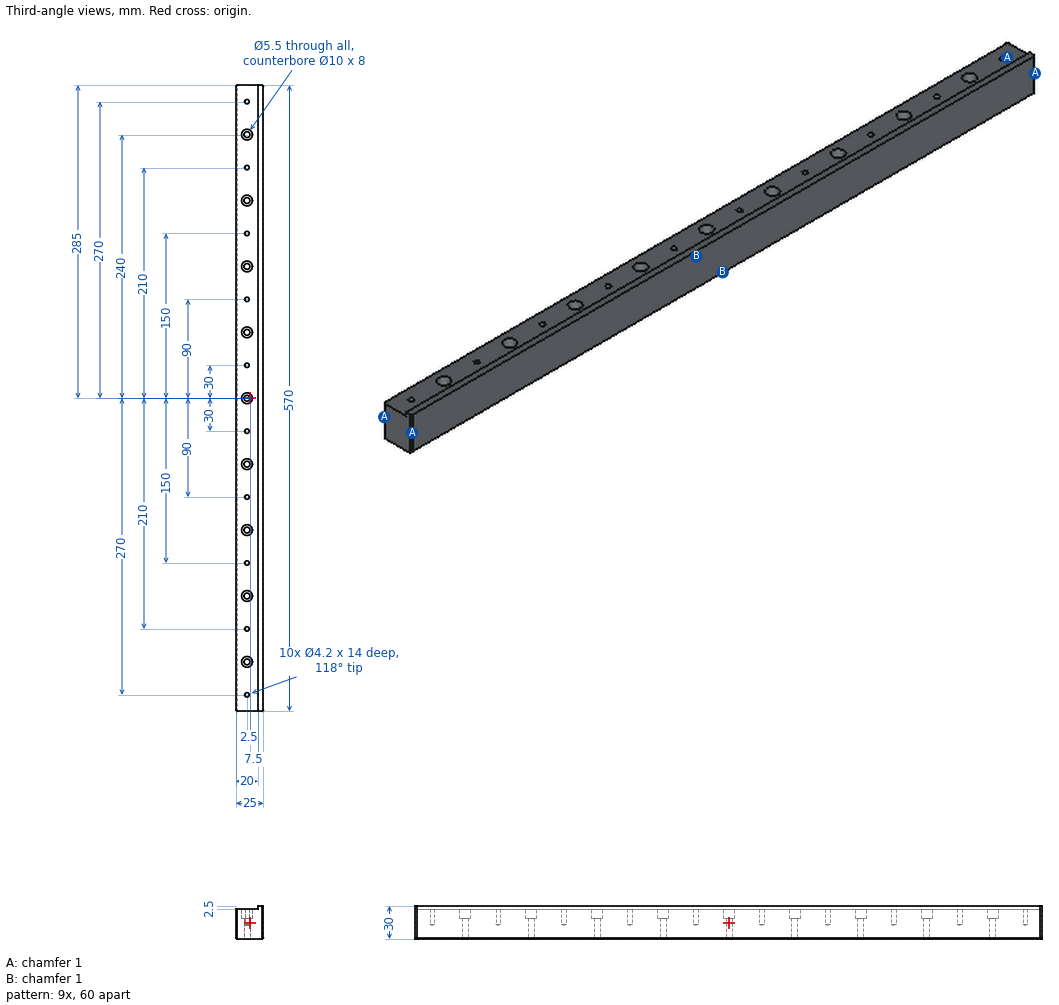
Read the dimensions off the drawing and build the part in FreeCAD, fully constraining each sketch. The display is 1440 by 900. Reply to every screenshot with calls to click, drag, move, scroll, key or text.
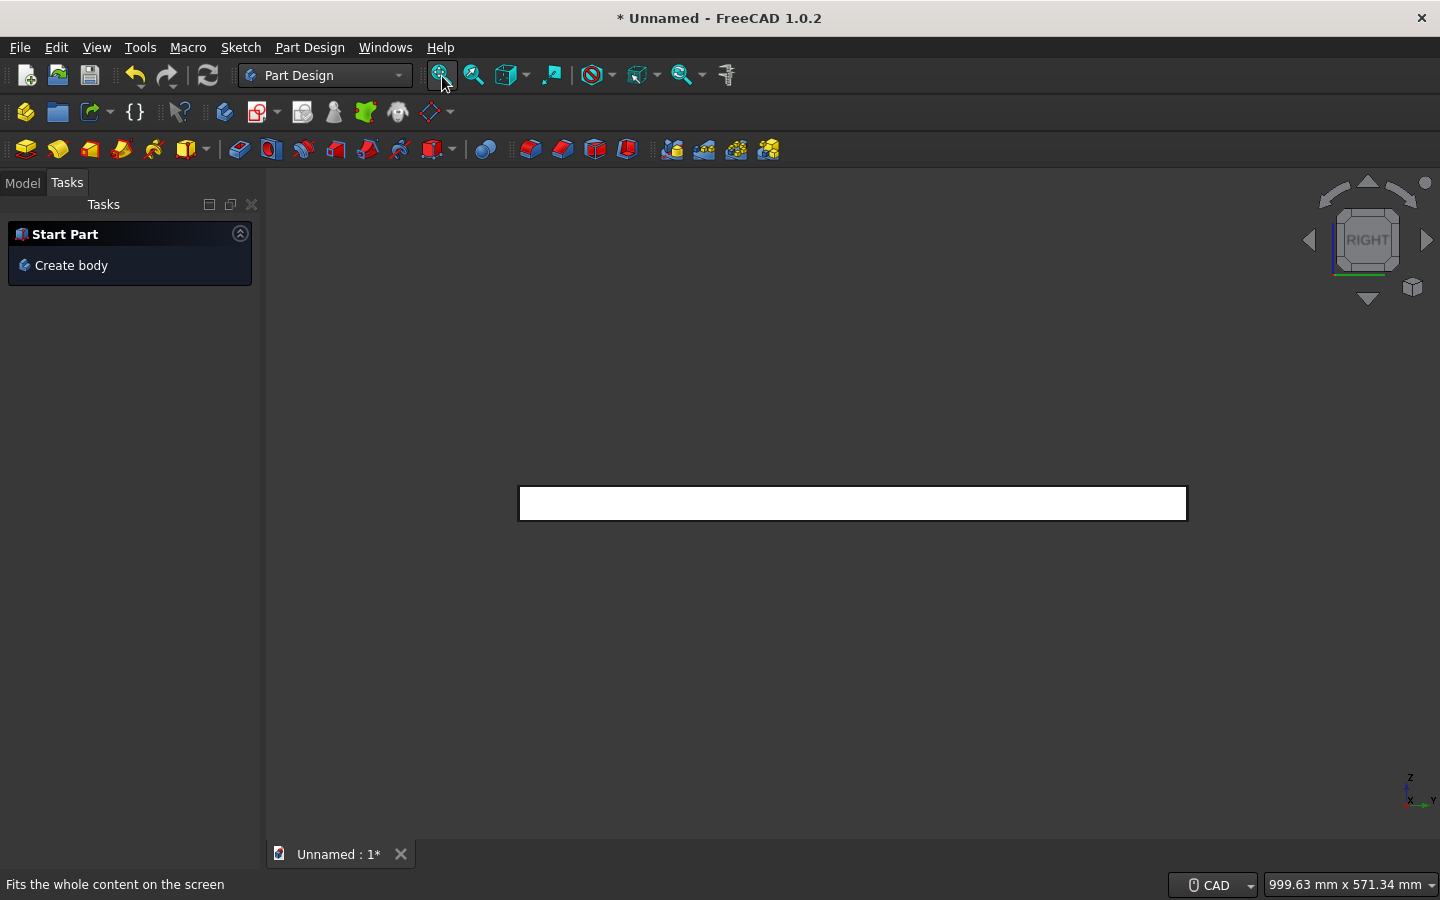
click(853, 520)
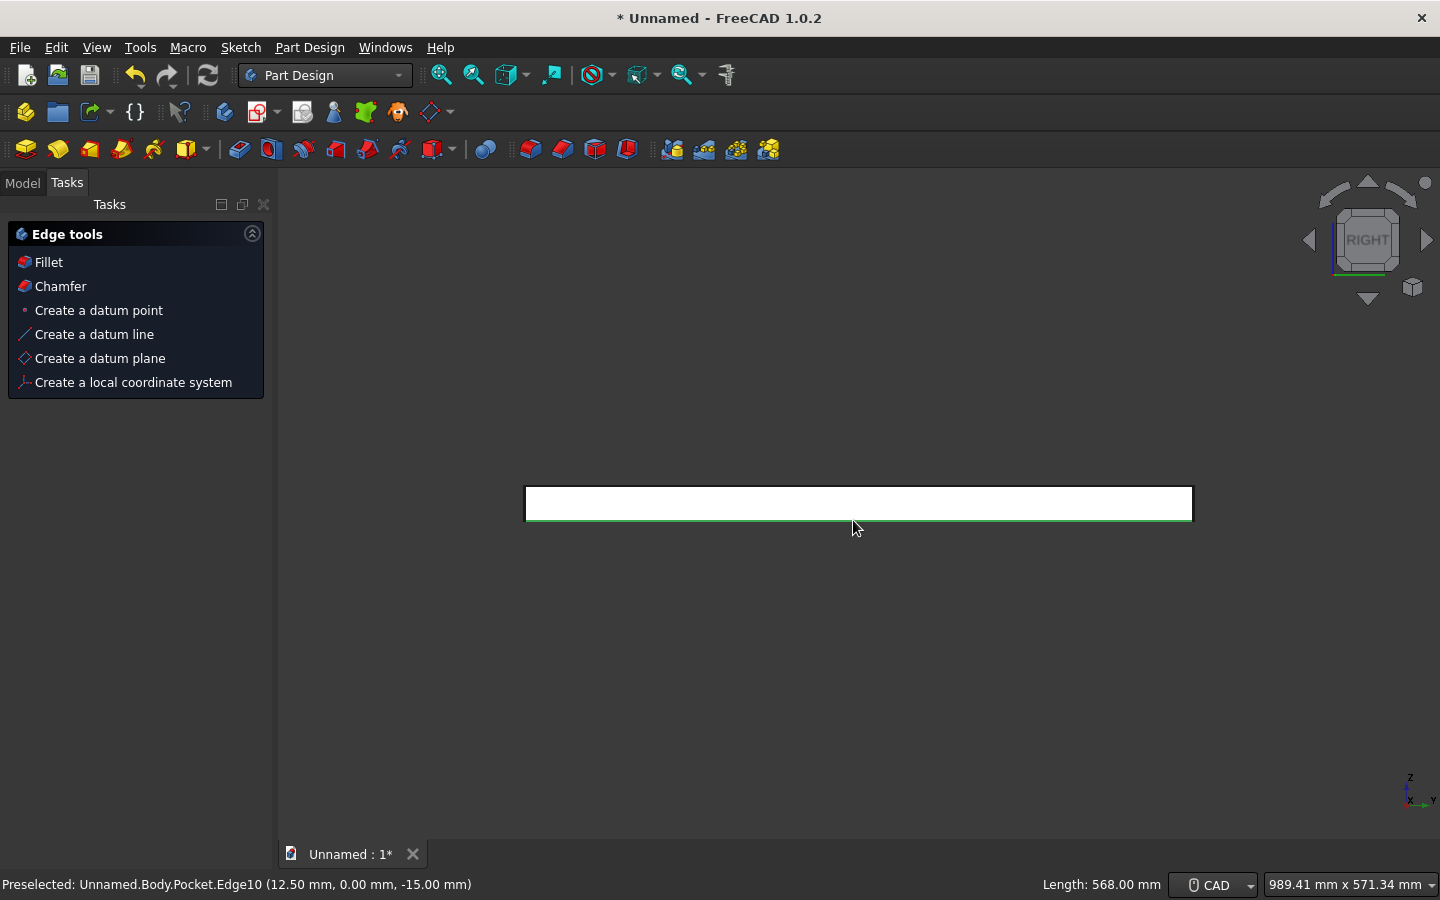
key(5)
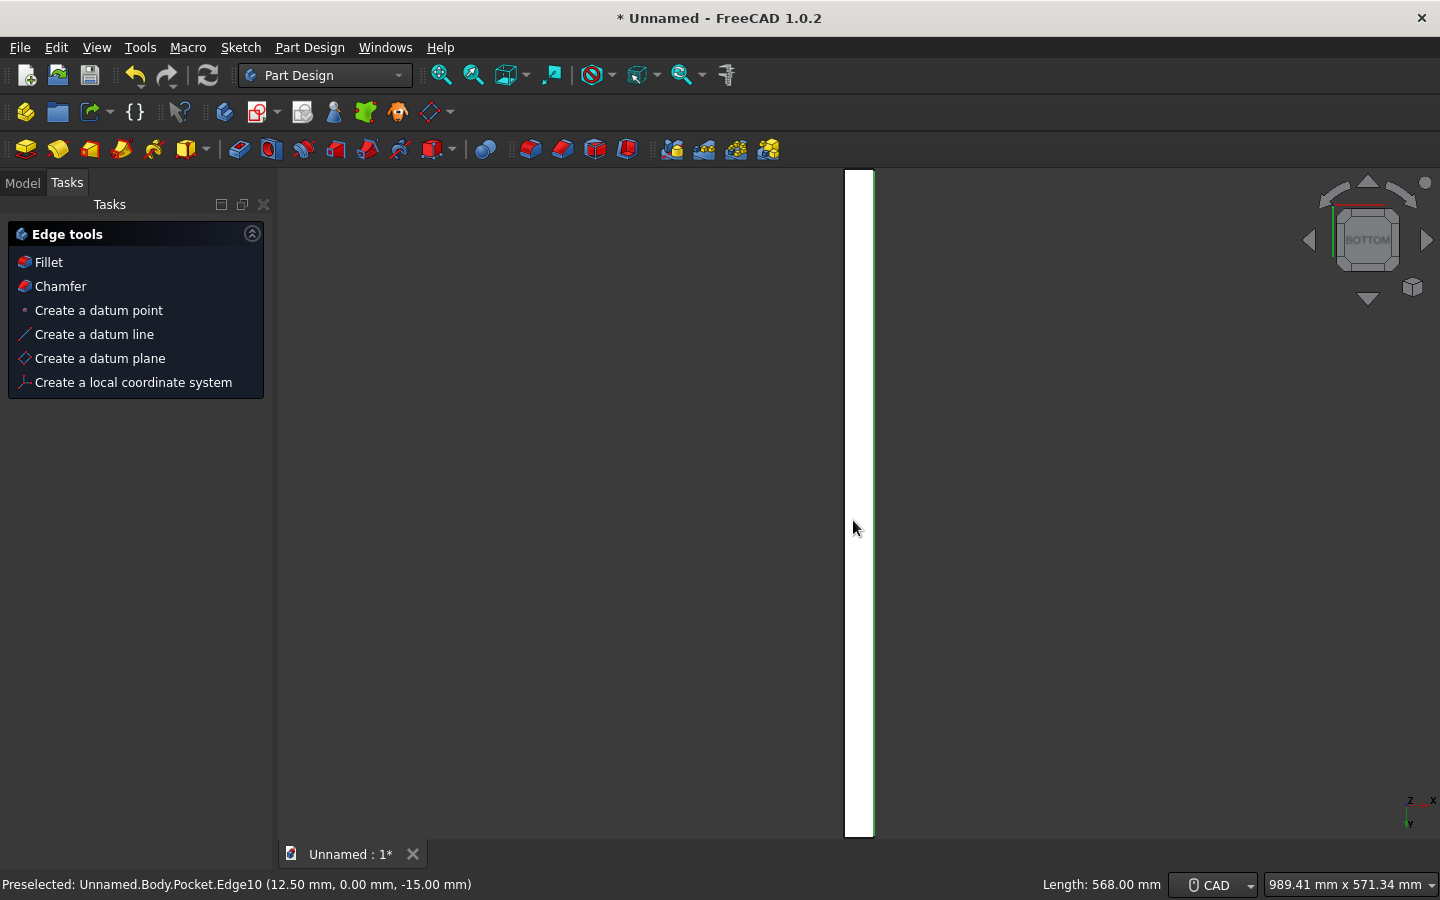
click(844, 502, ctrl)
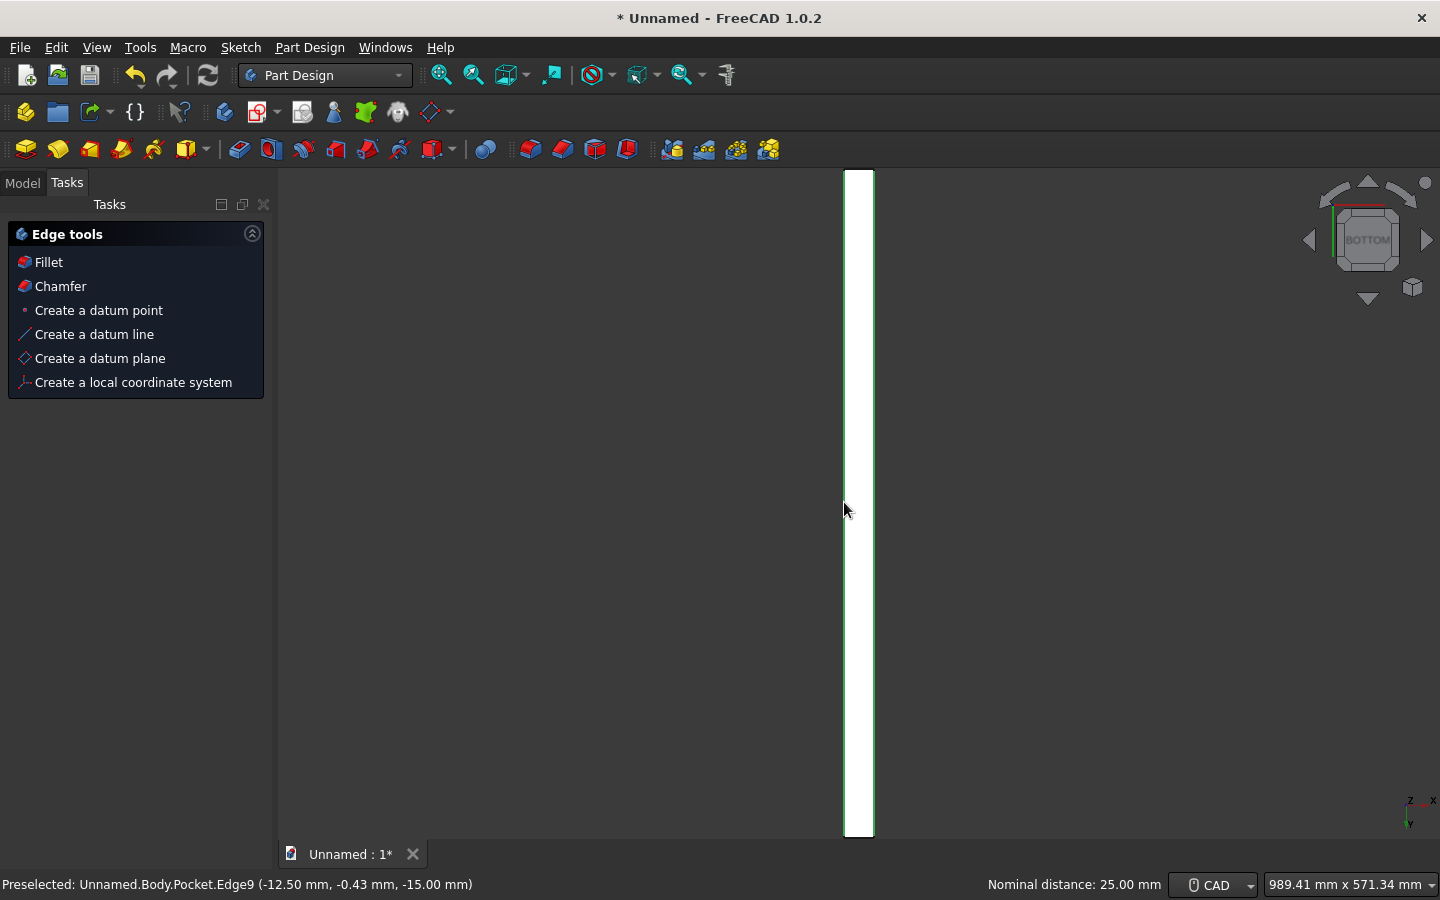
click(564, 150)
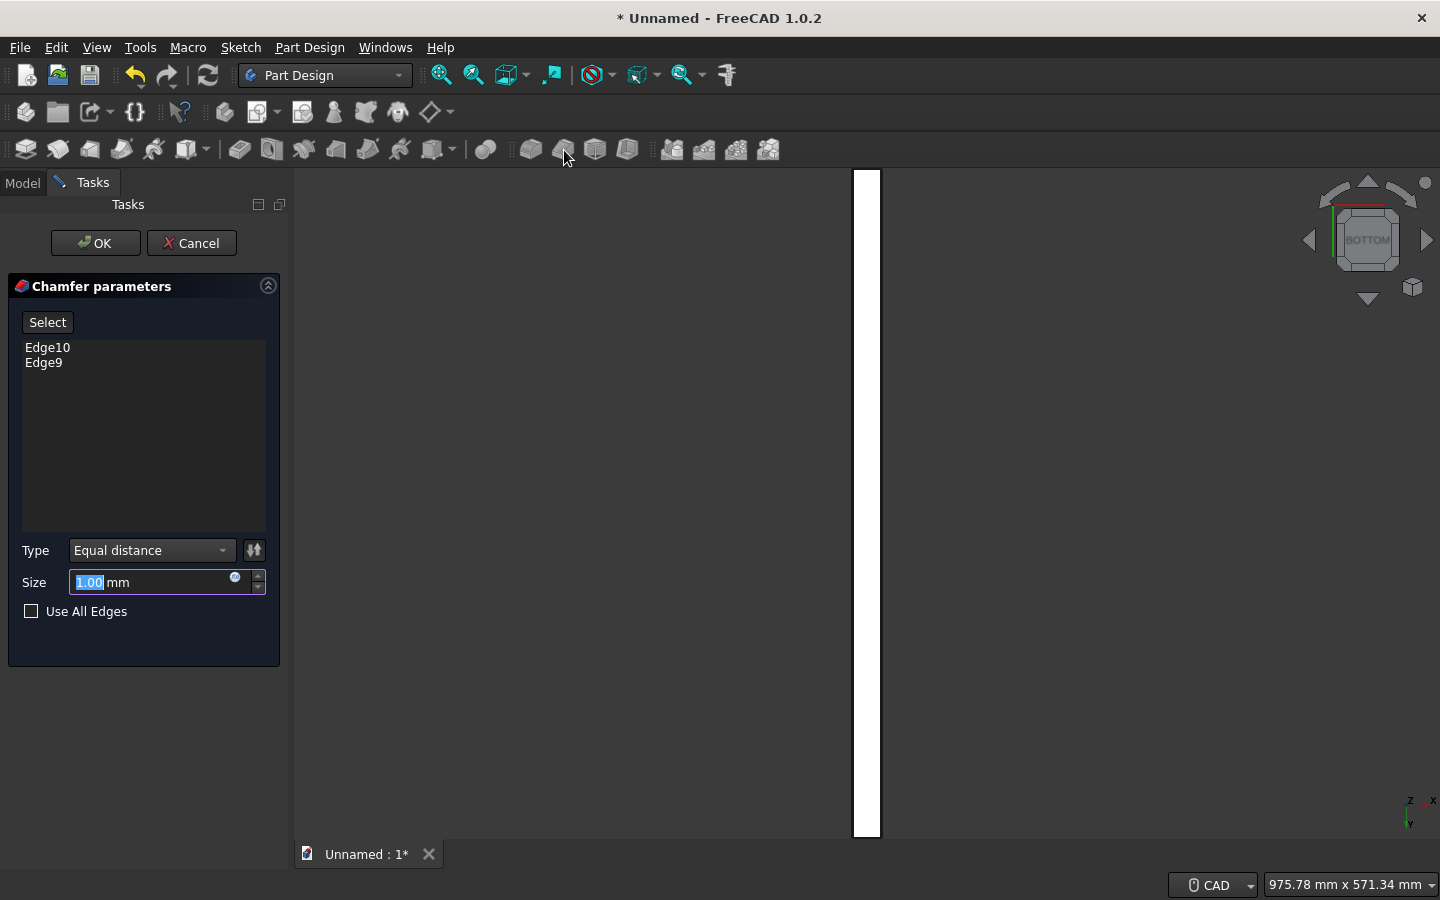
text(1)
key(Tab)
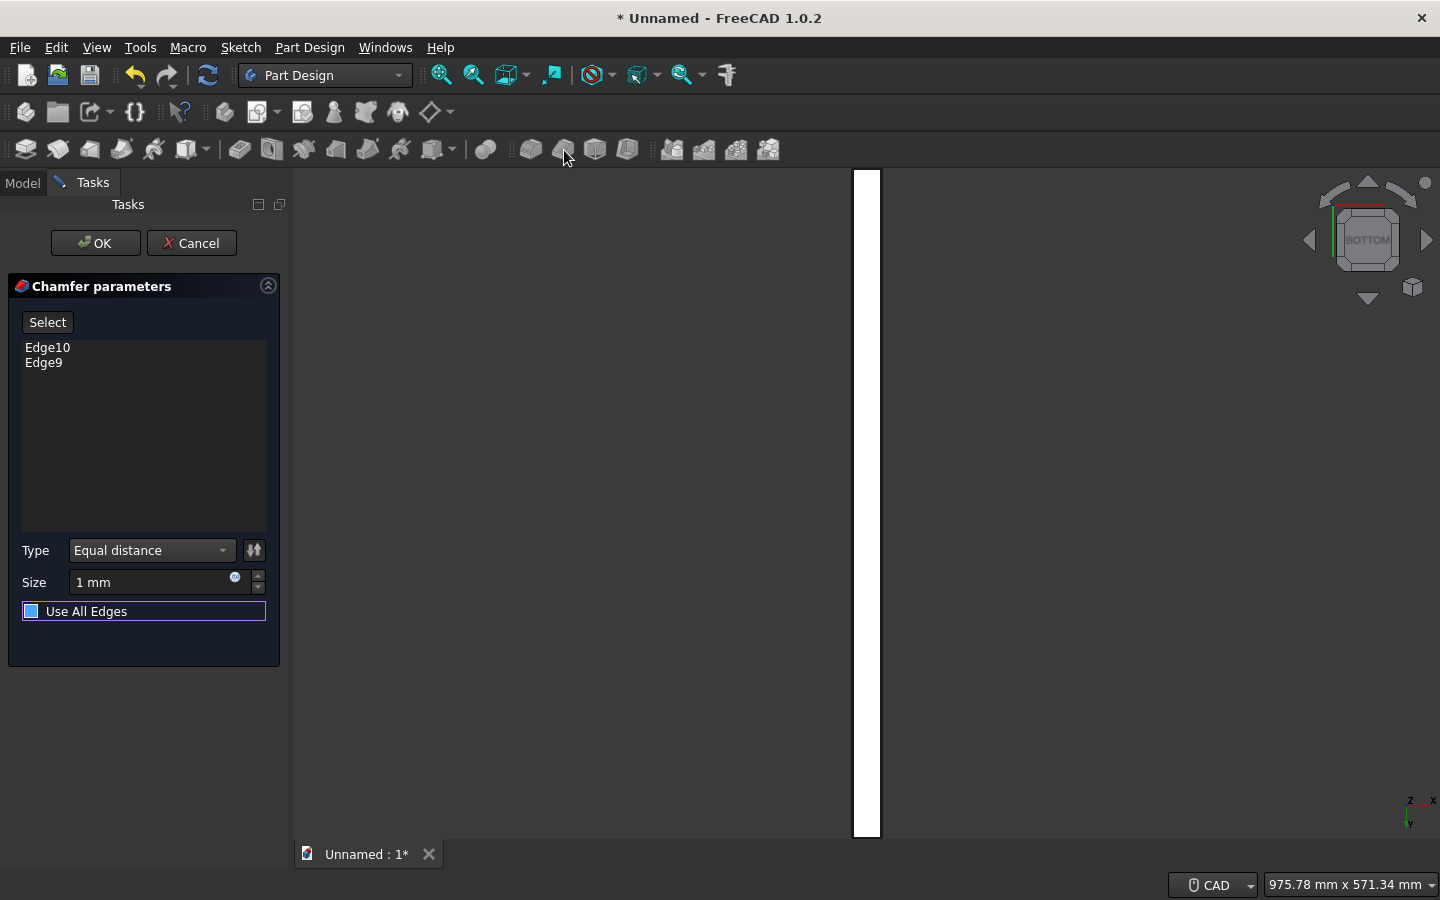
click(96, 243)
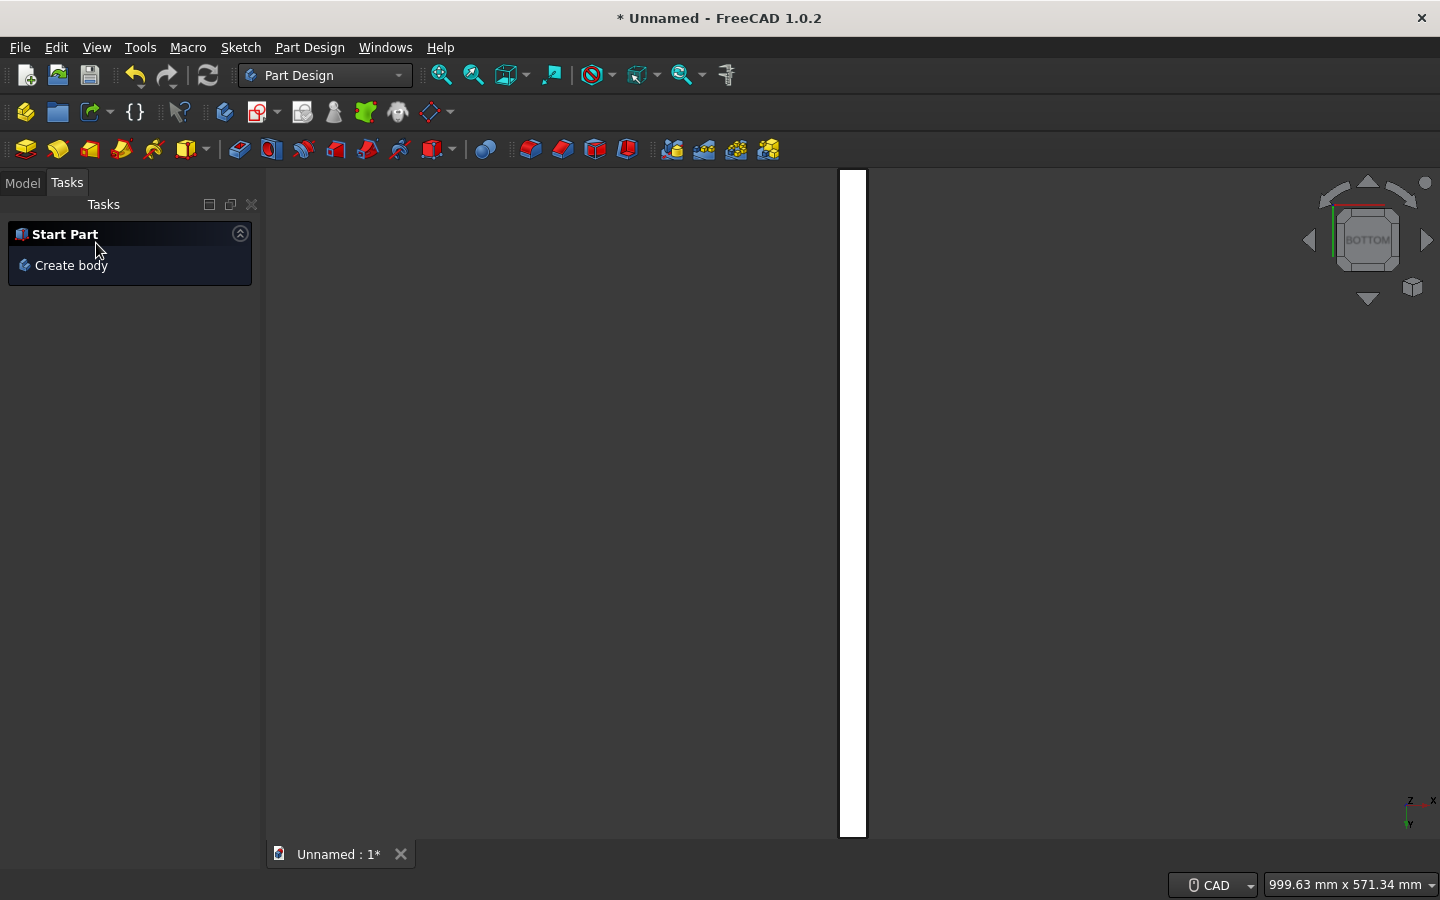
key(0)